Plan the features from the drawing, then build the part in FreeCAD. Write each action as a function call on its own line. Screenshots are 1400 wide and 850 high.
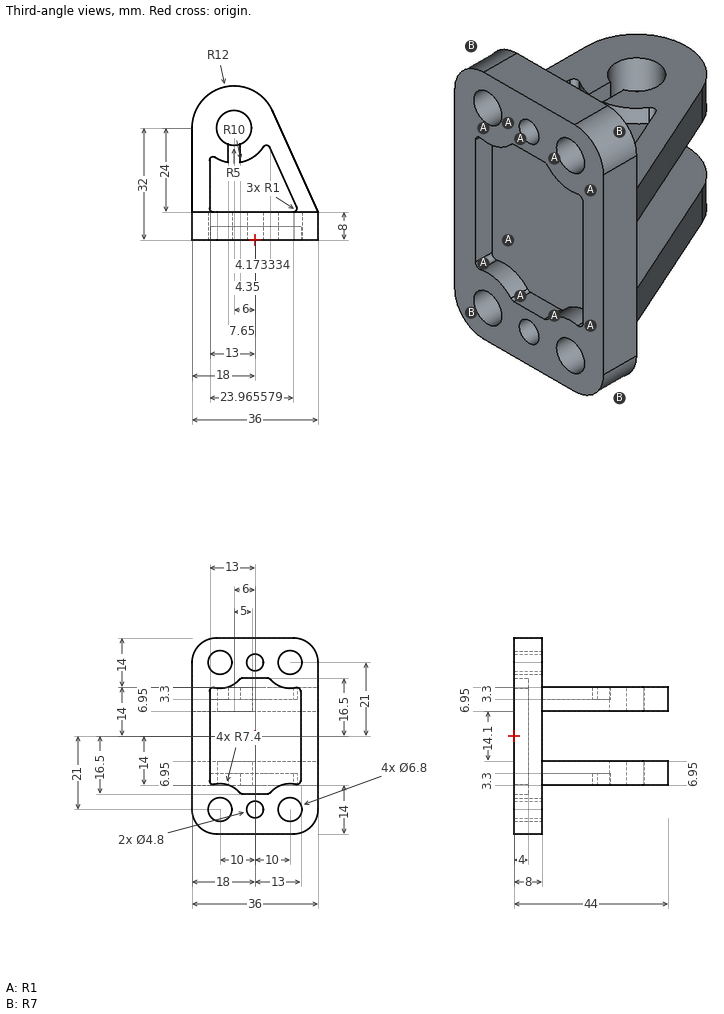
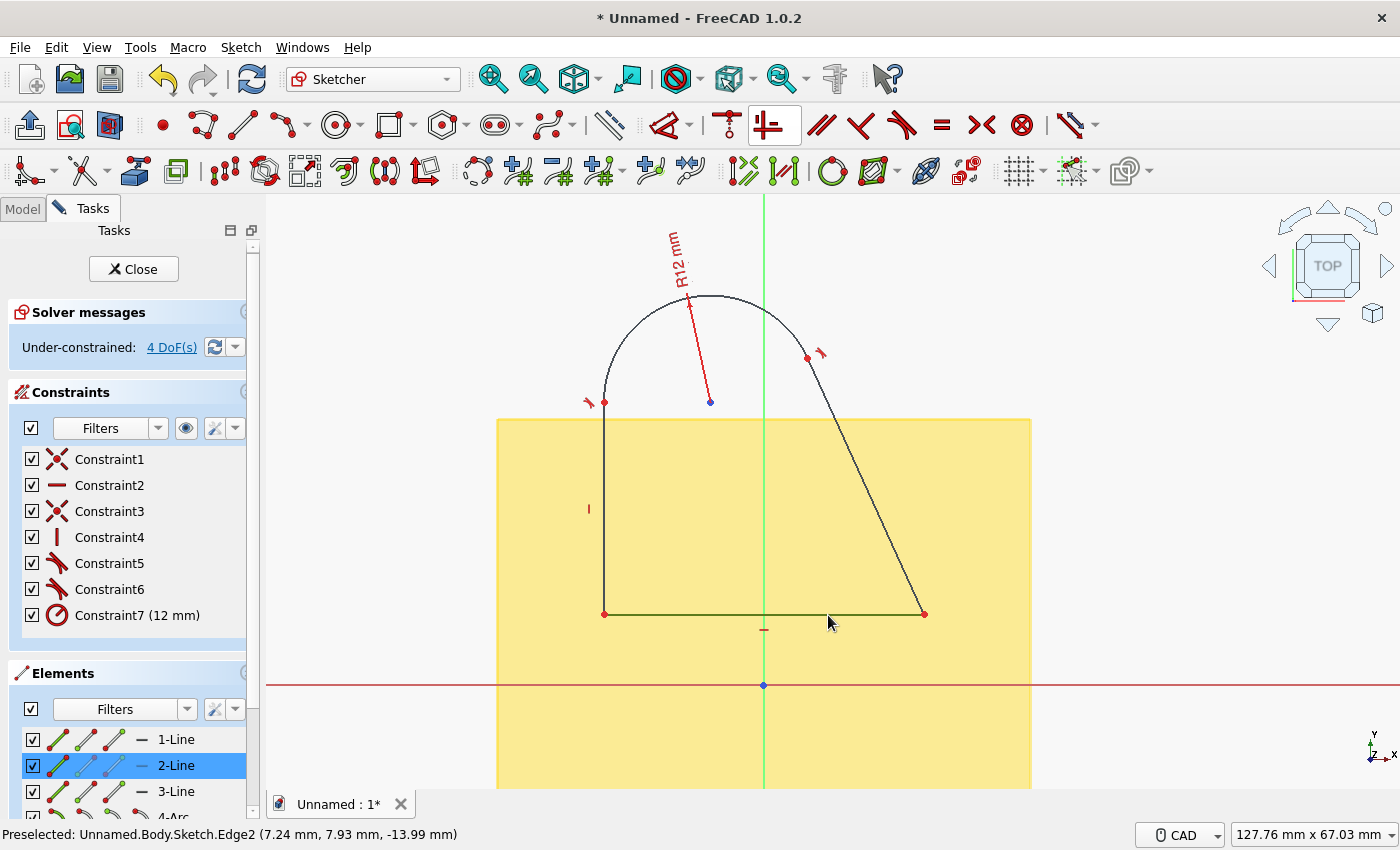
key(l)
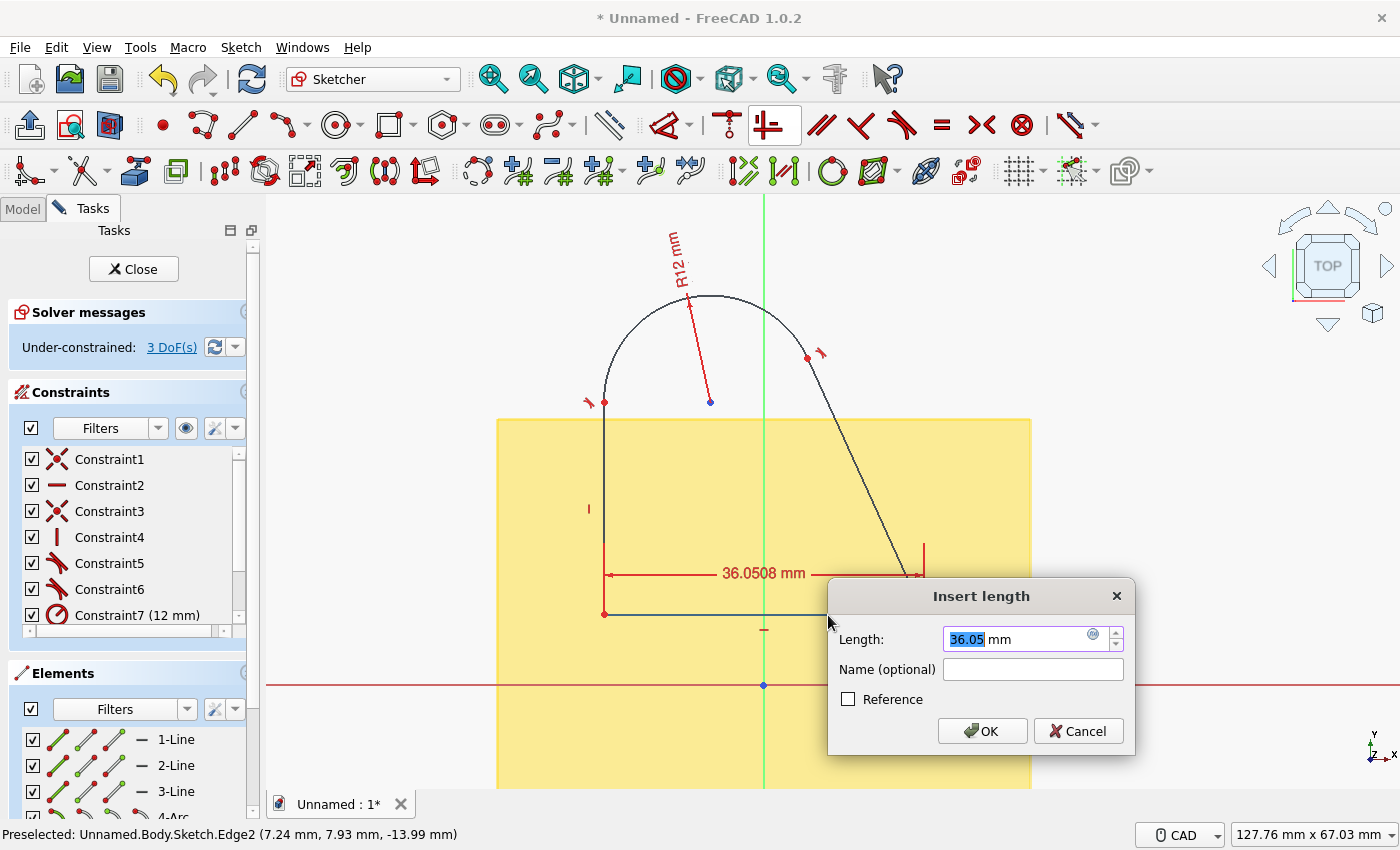
text(36)
key(Return)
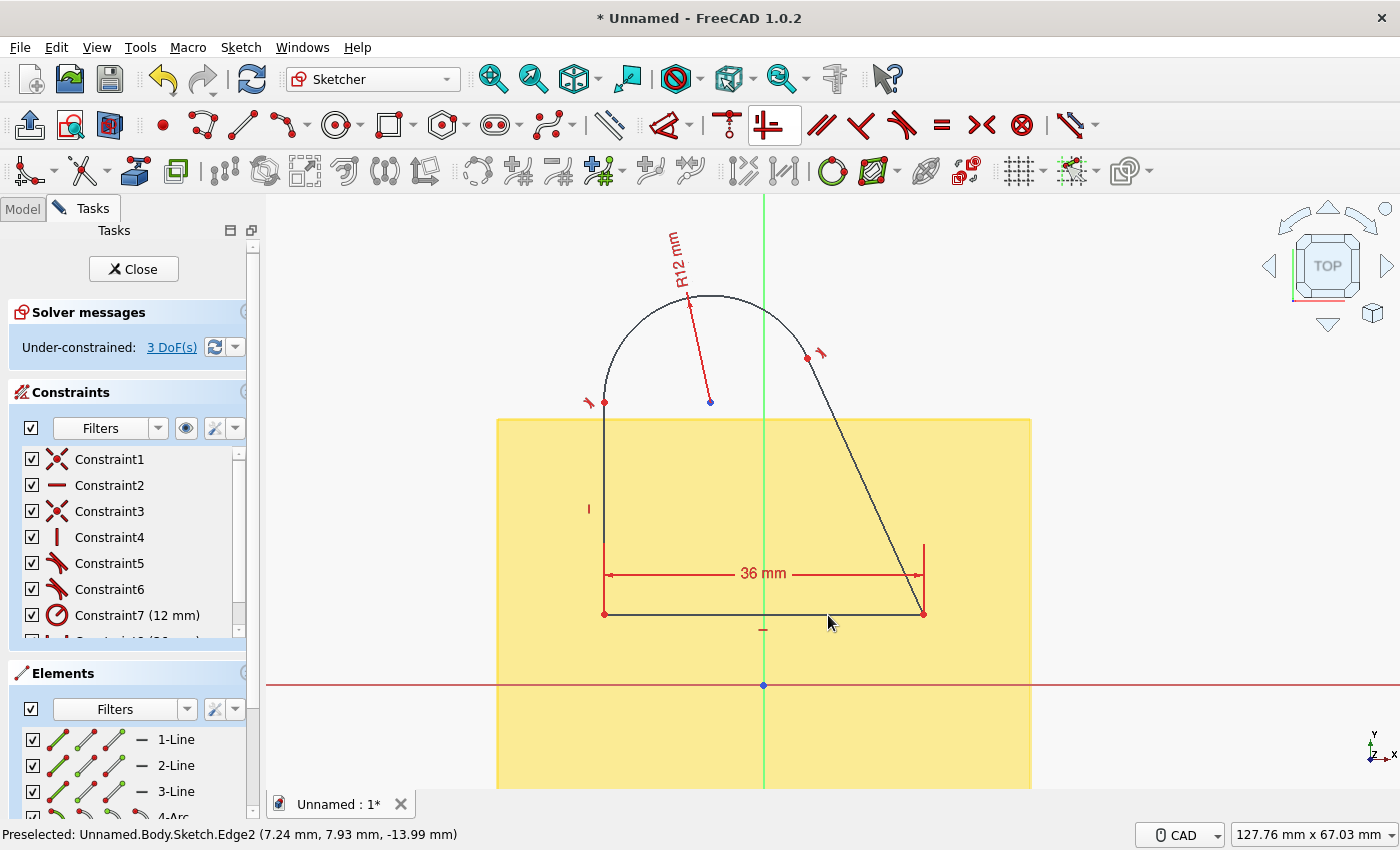
click(604, 551)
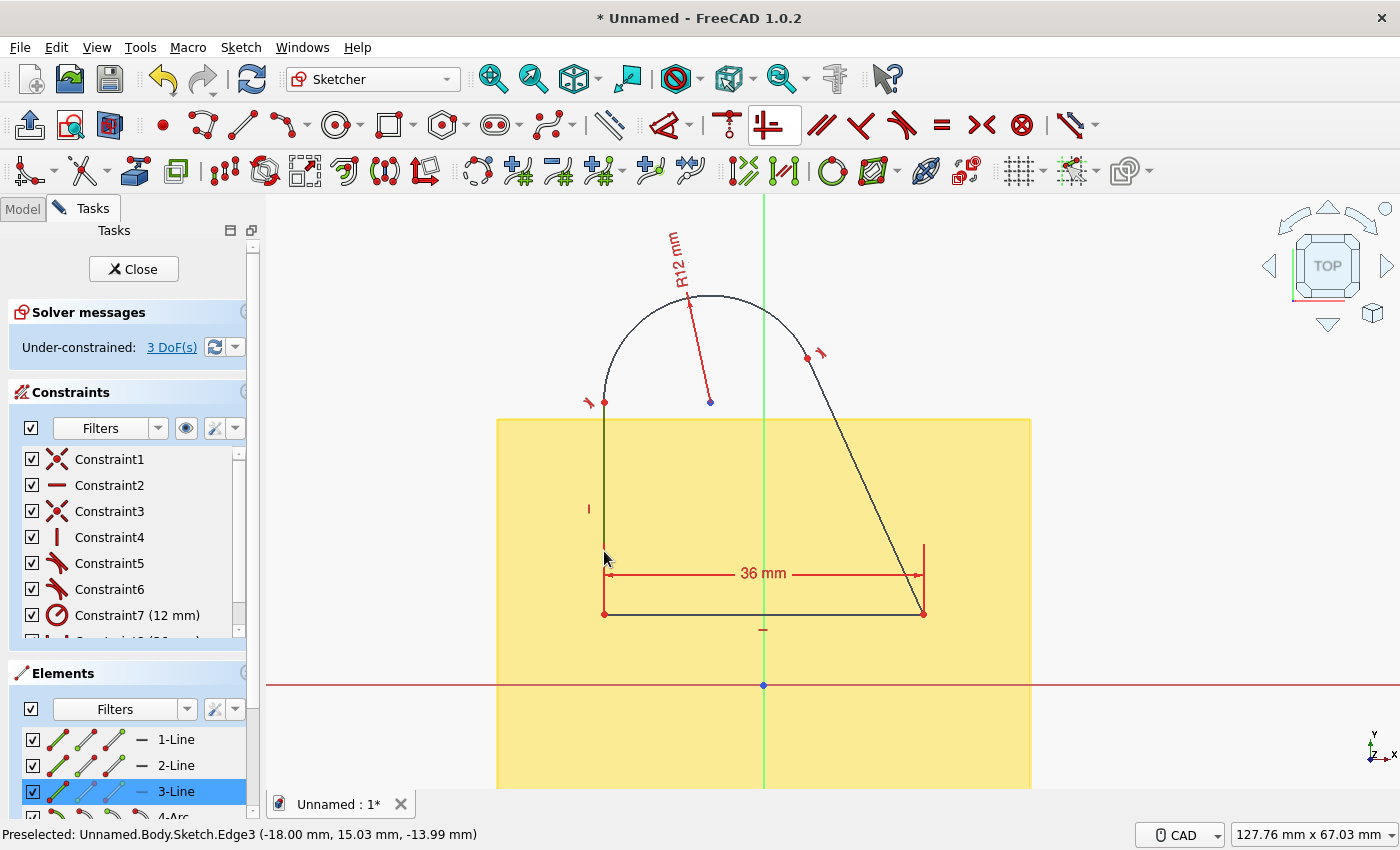
key(i)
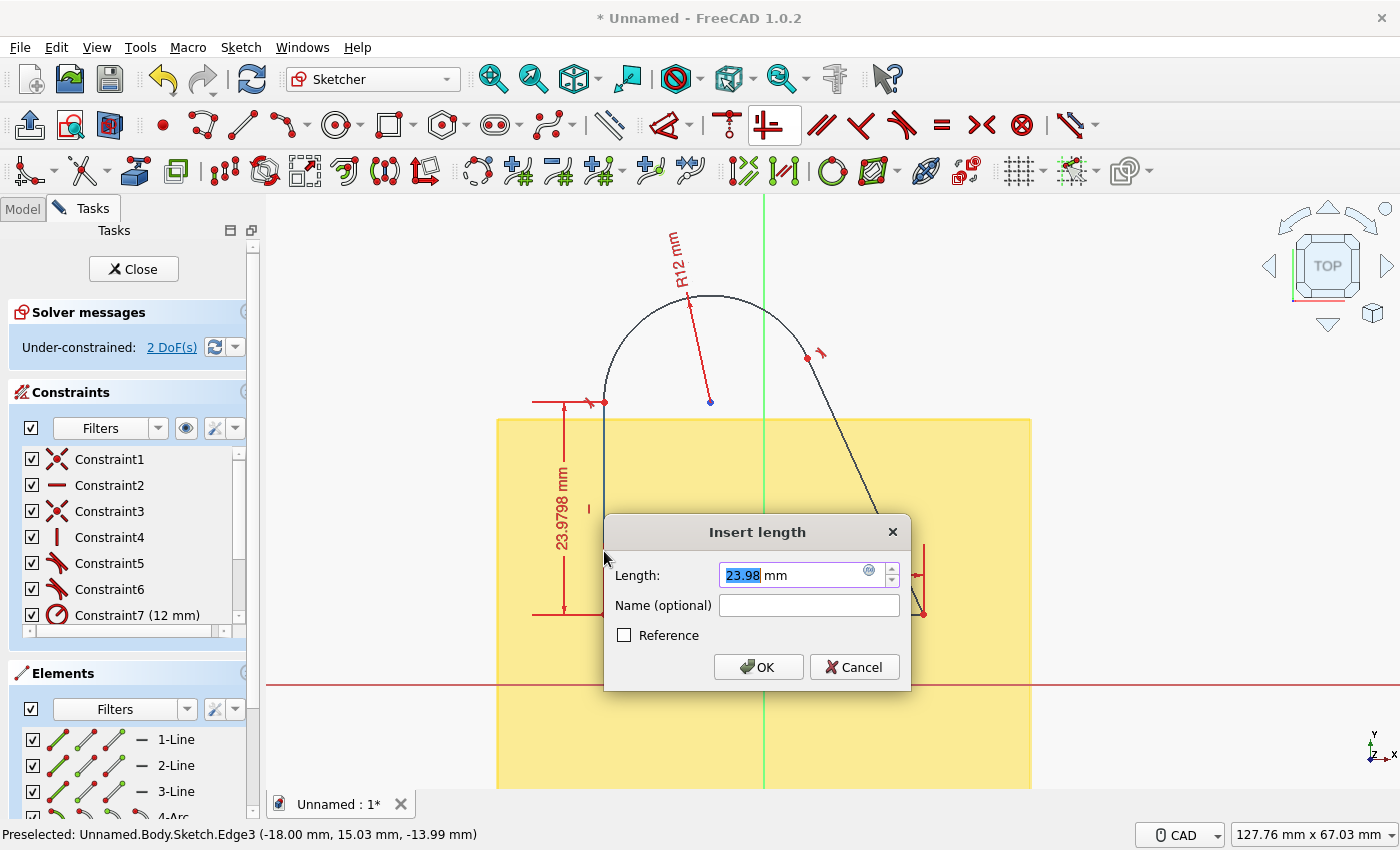
text(24)
key(Return)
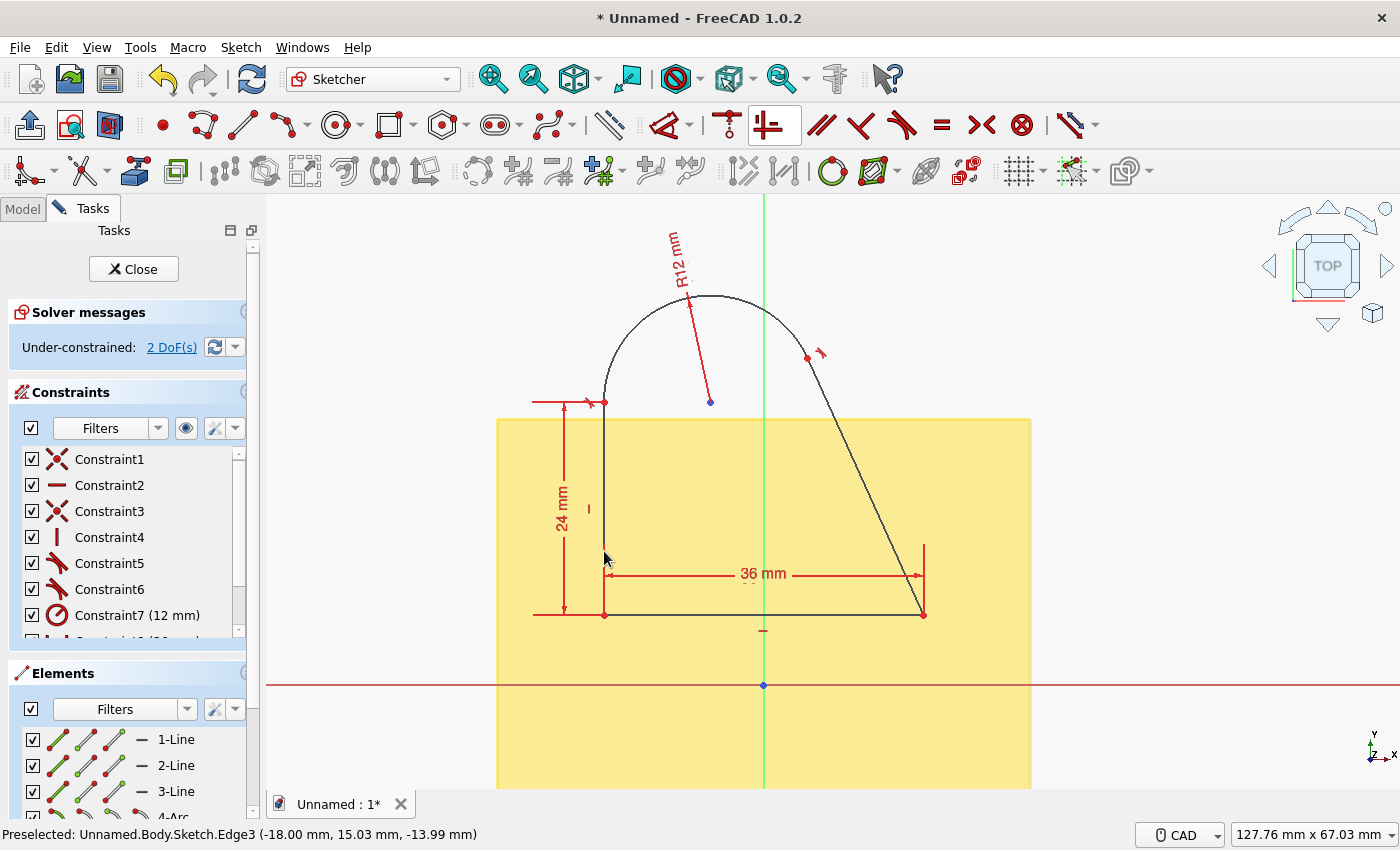
click(924, 615)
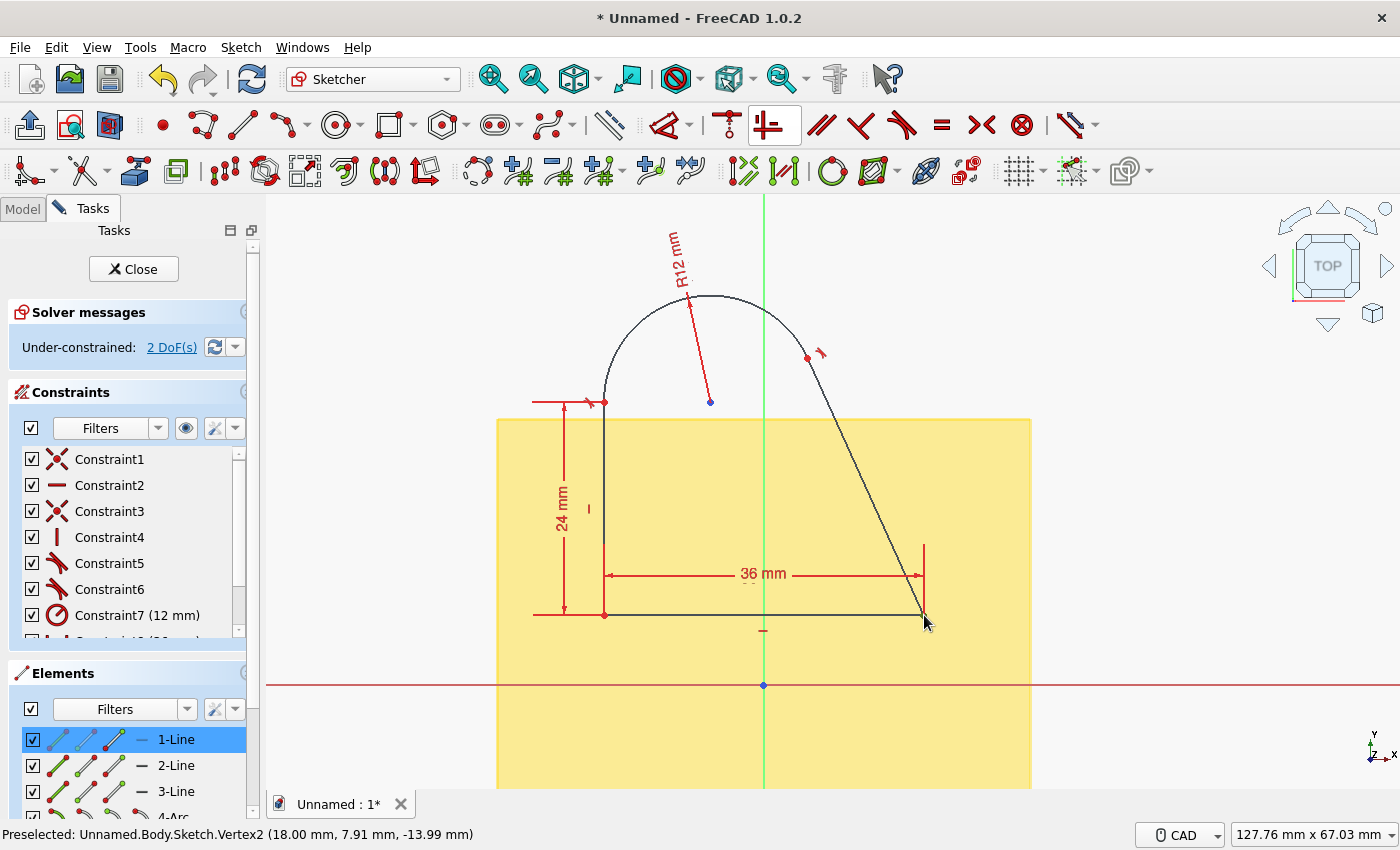
key(i)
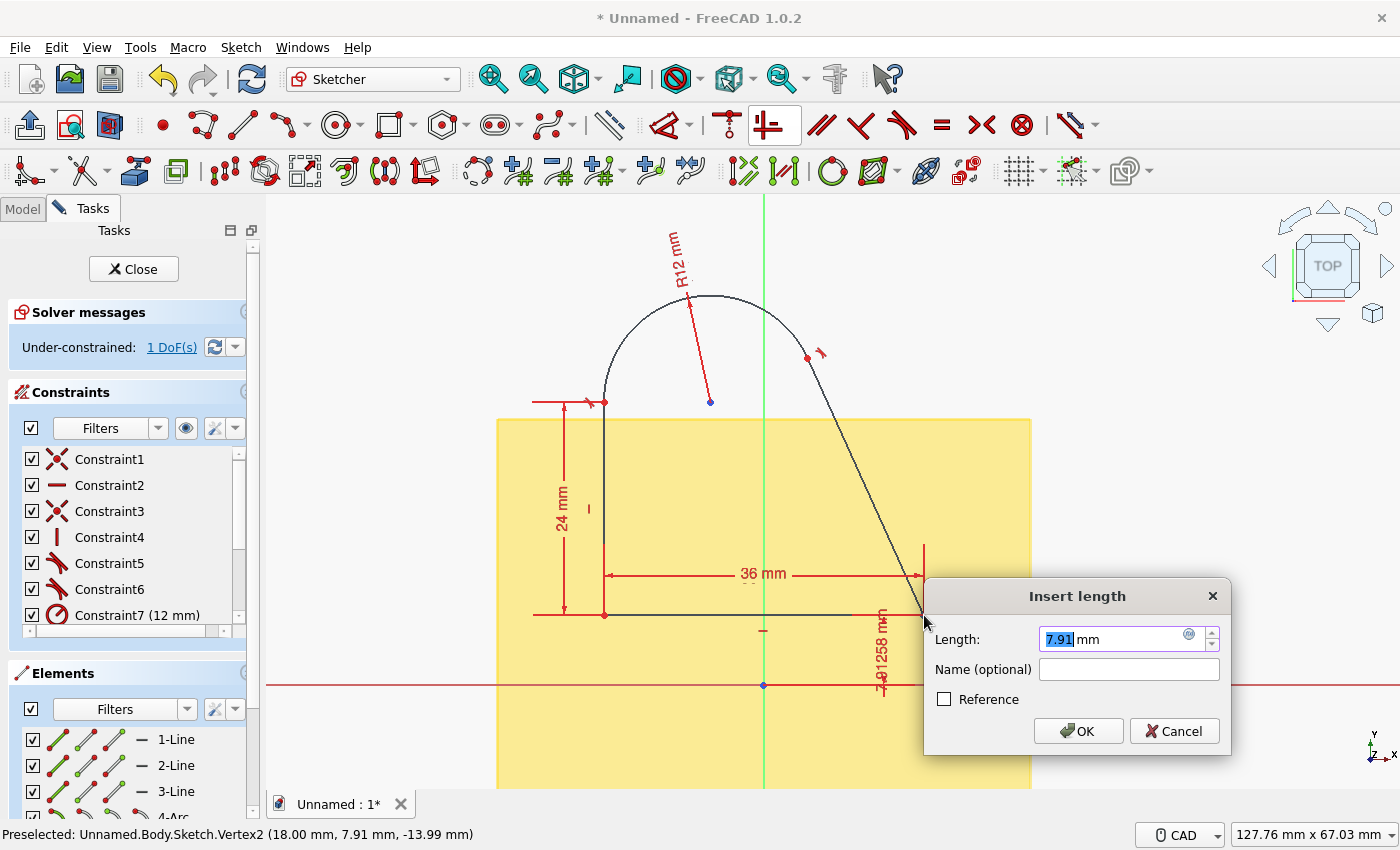
text(8)
key(Return)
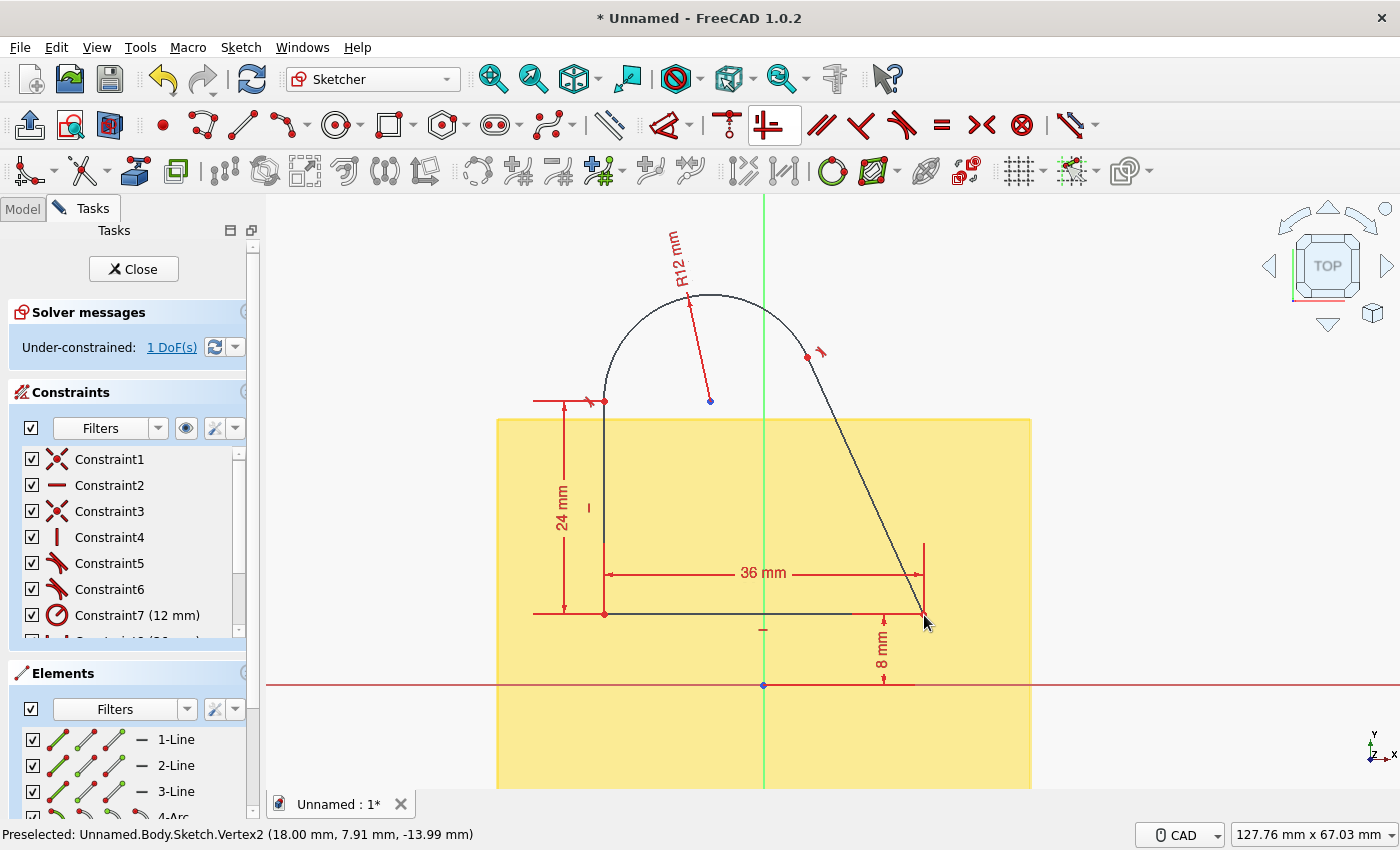
click(711, 401)